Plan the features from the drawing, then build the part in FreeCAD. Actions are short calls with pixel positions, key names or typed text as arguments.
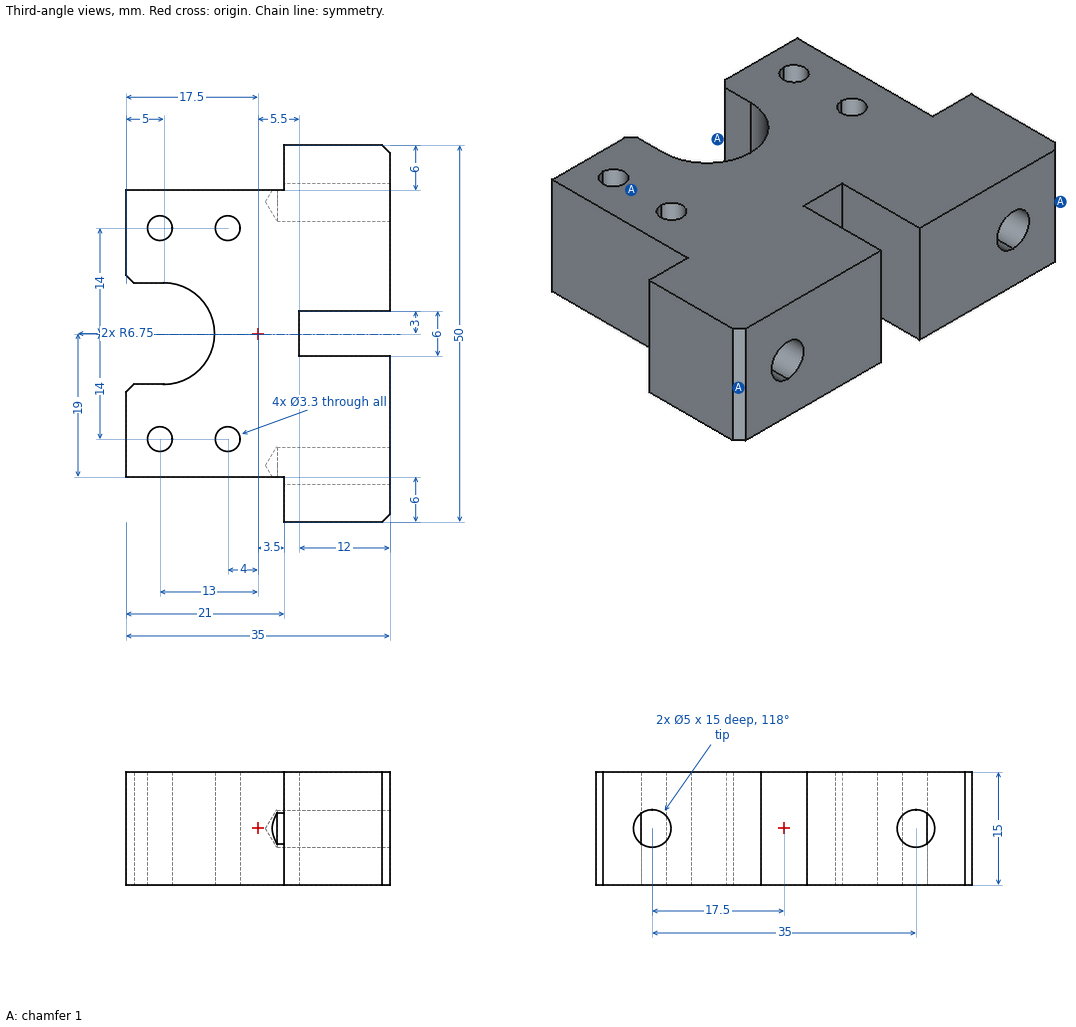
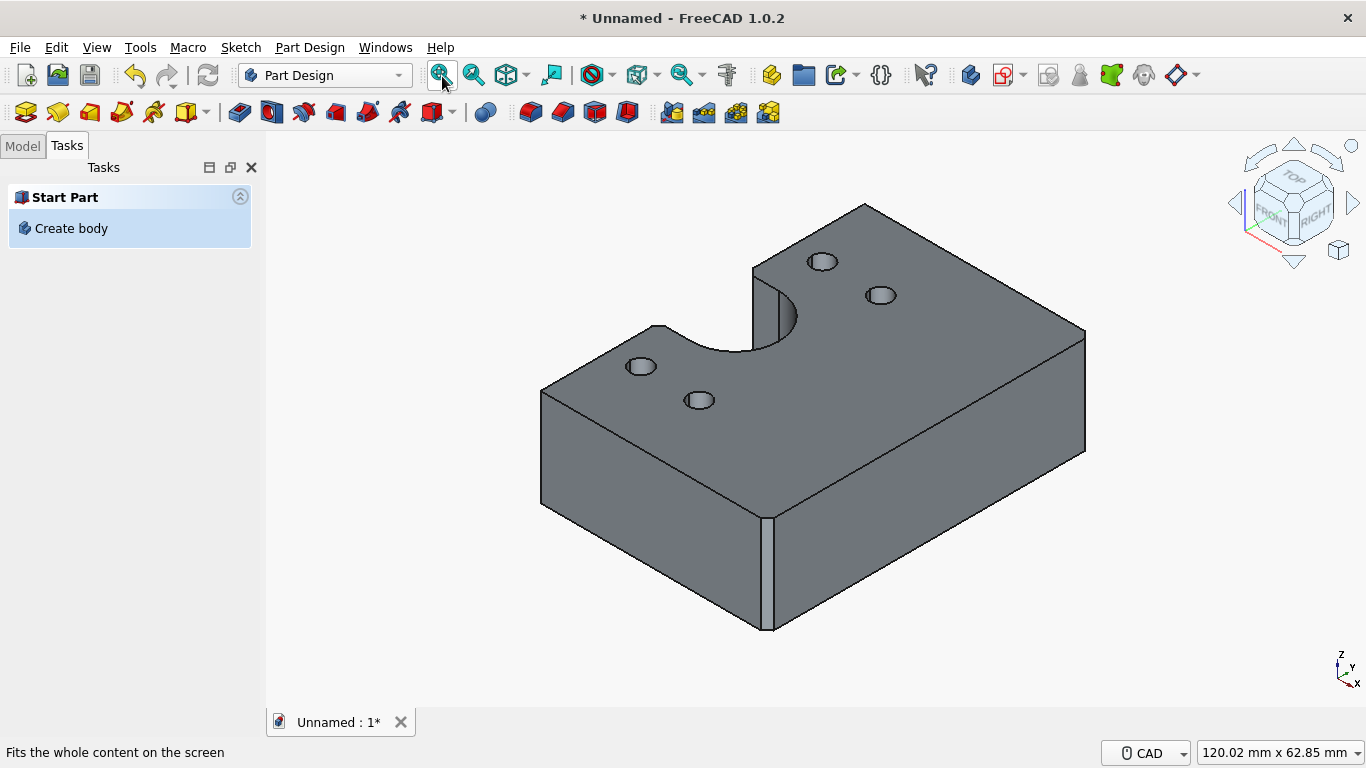
click(1018, 432)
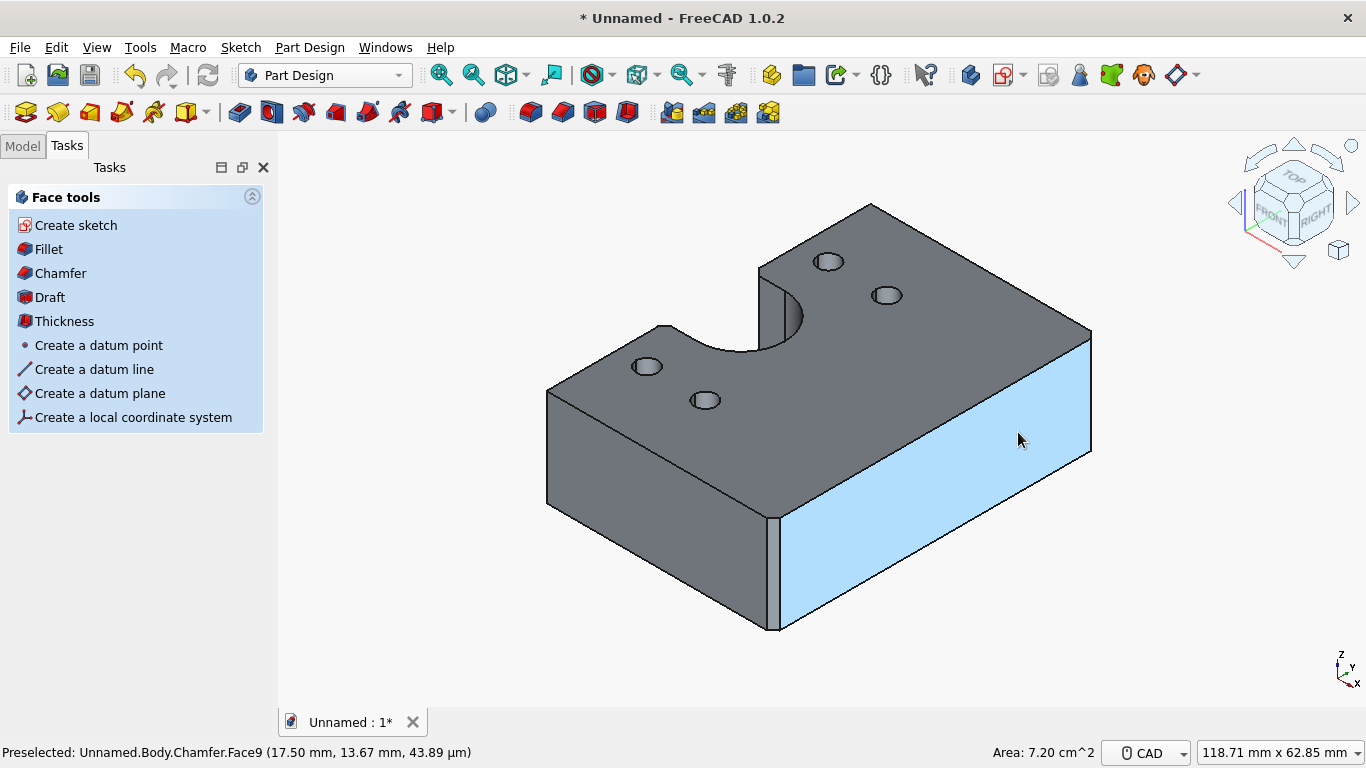
click(1004, 76)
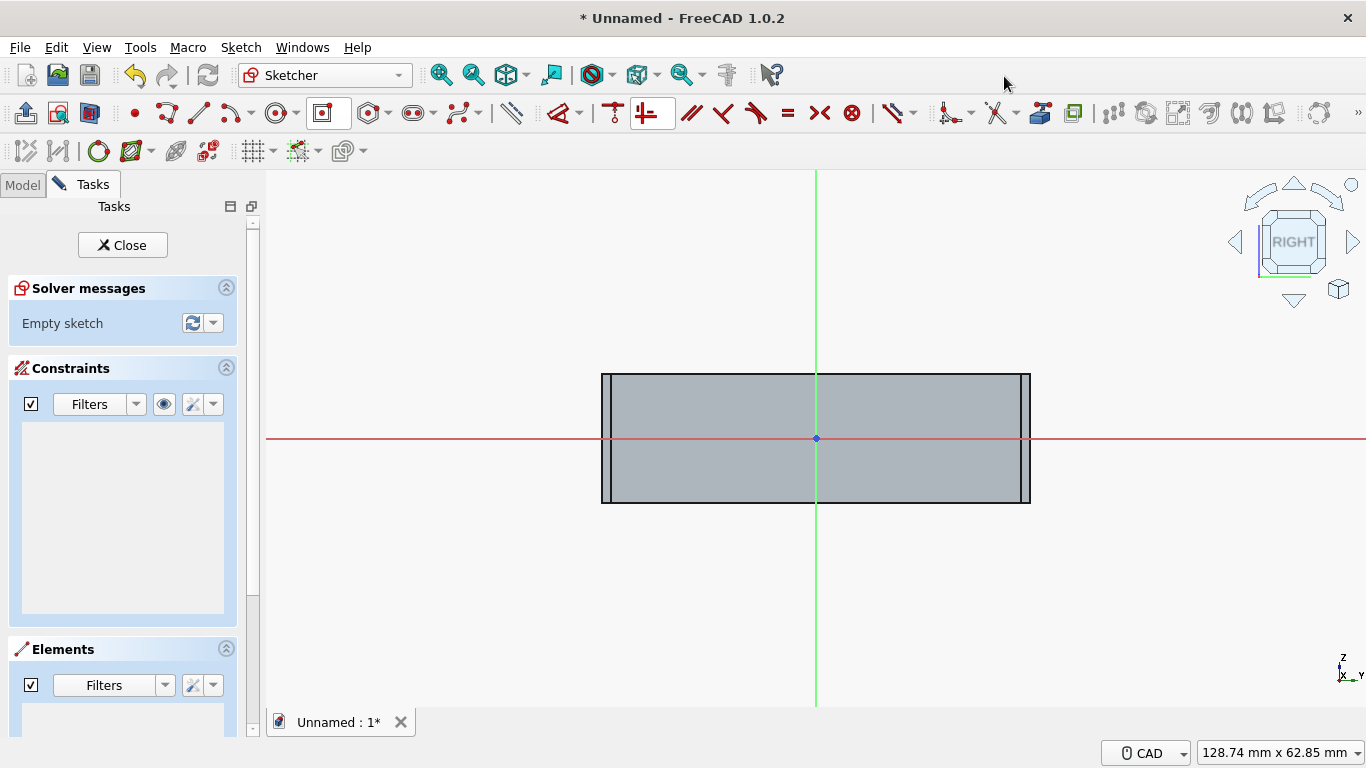
scroll(899, 438, up, 3)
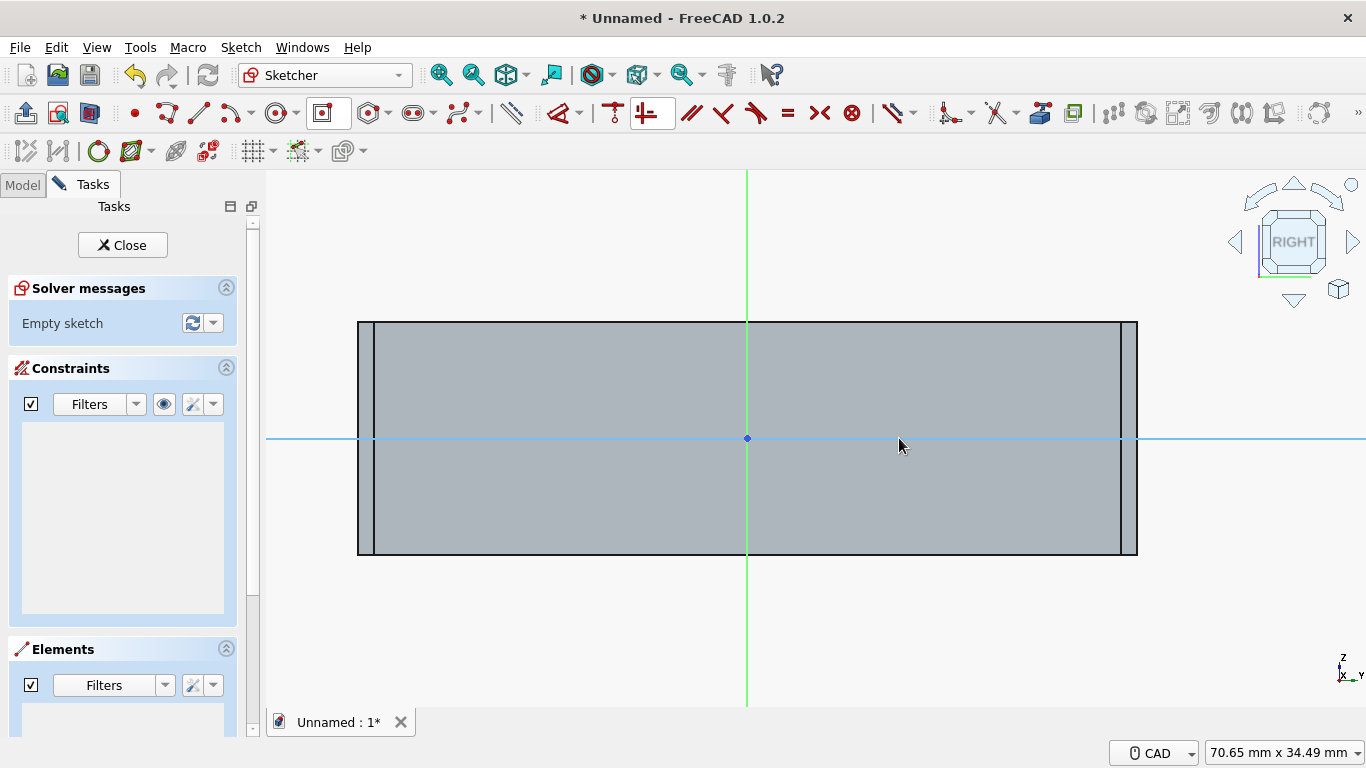
click(276, 114)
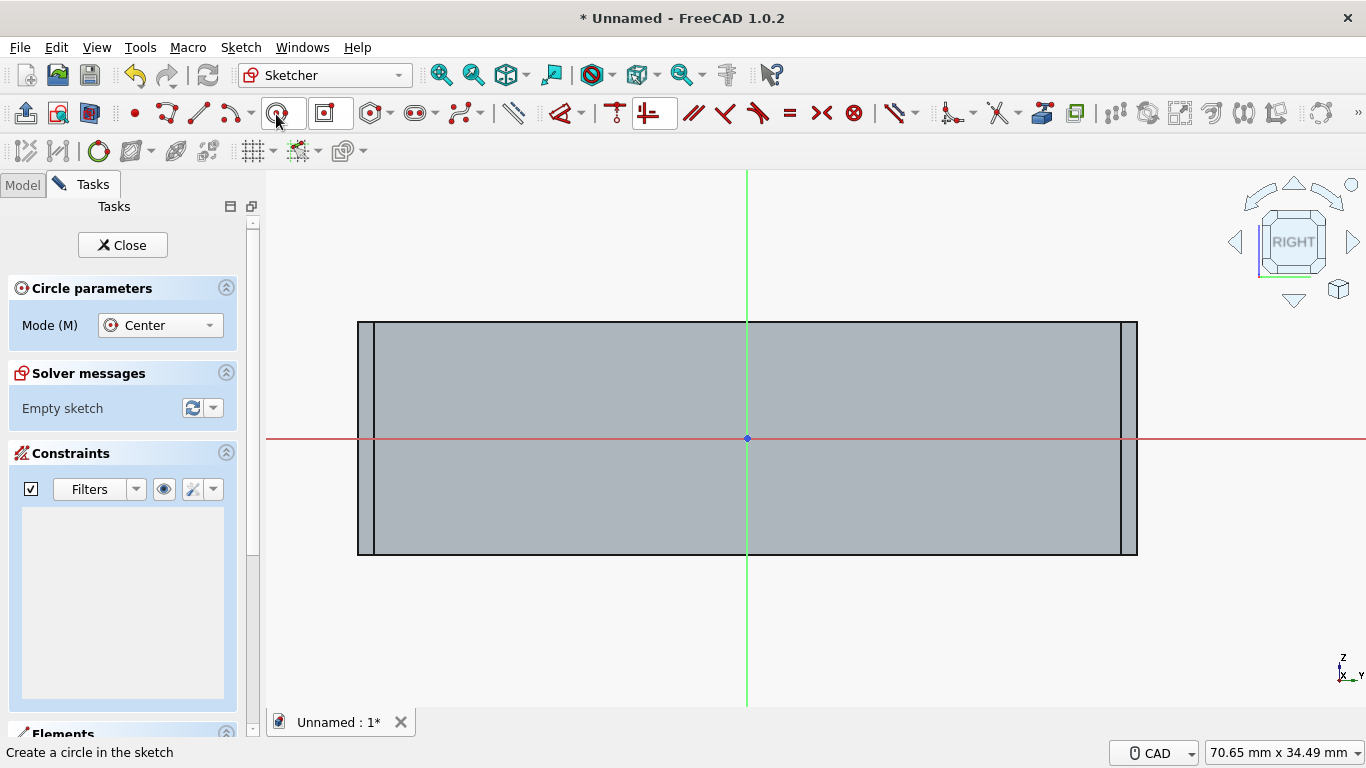
click(475, 438)
move(502, 411)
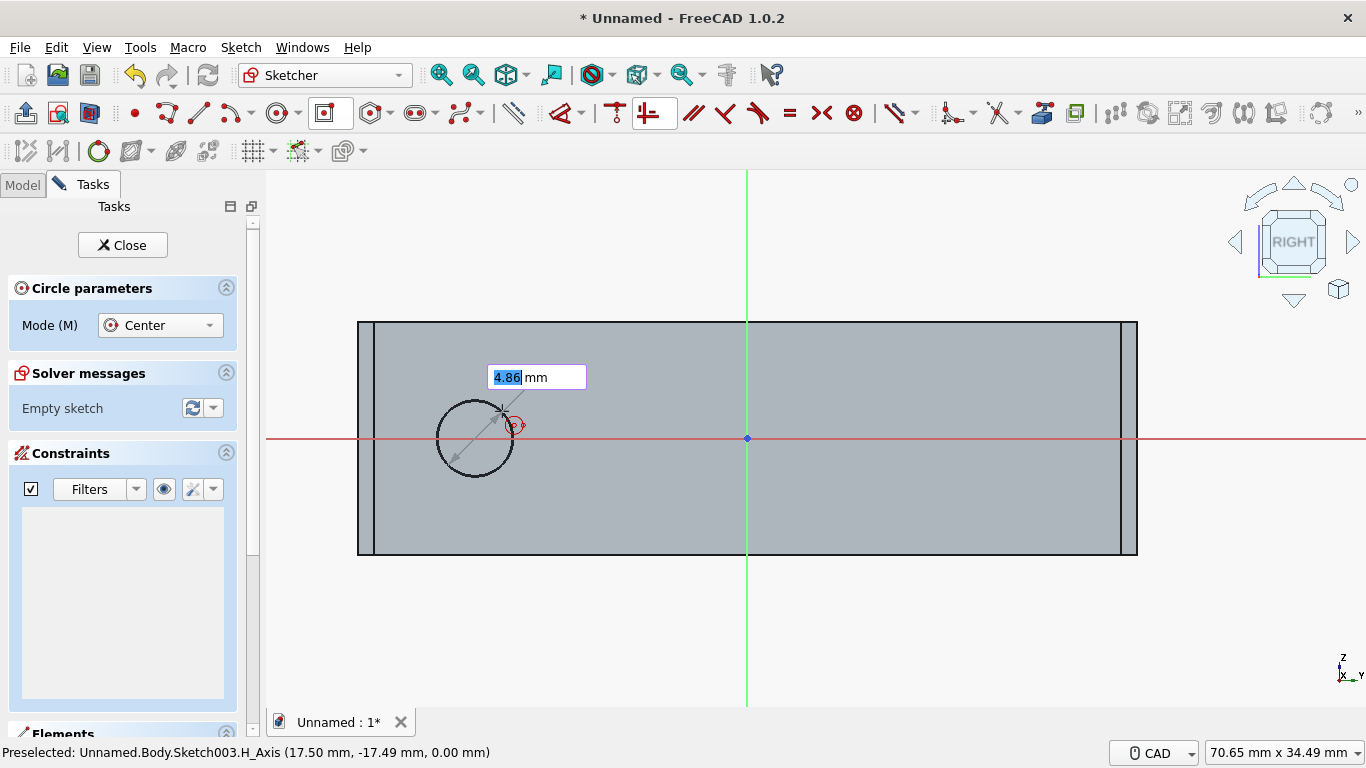
text(5)
key(Return)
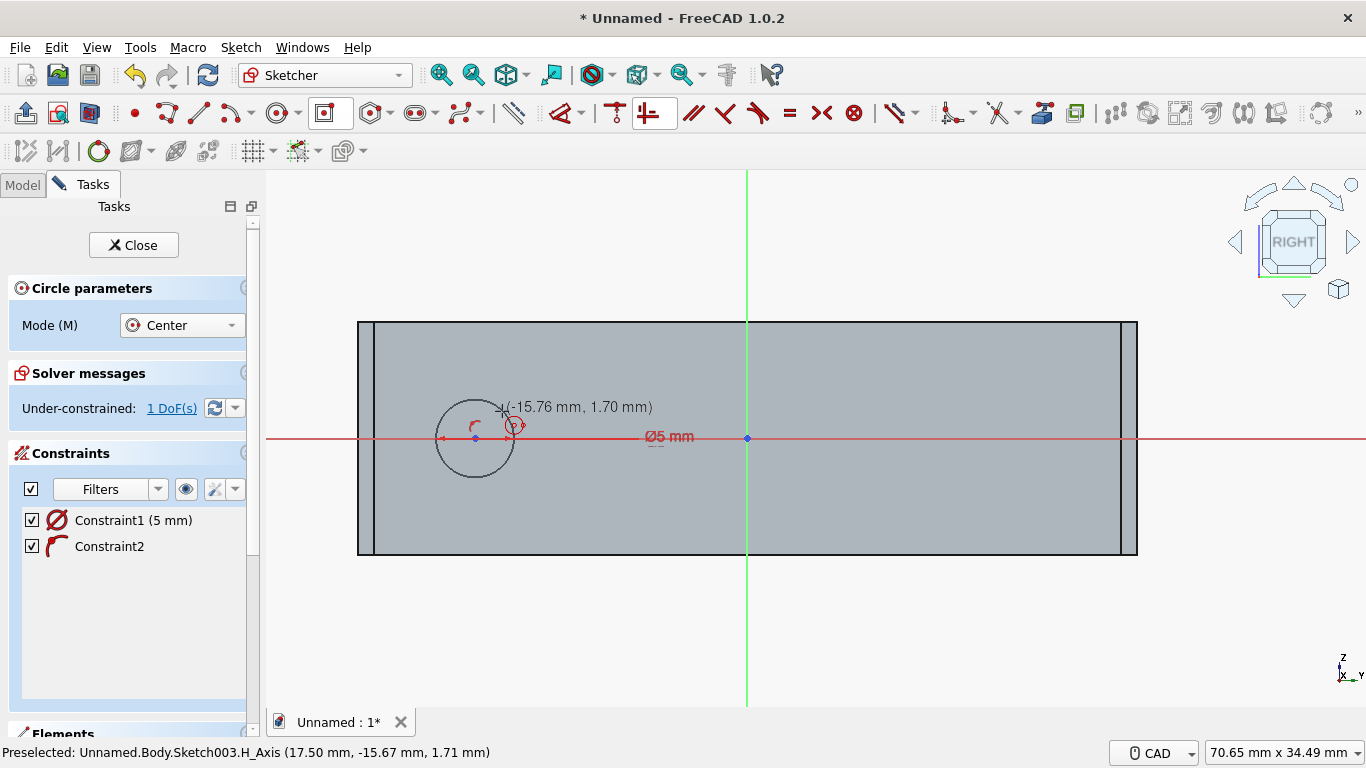
click(1020, 438)
move(1047, 411)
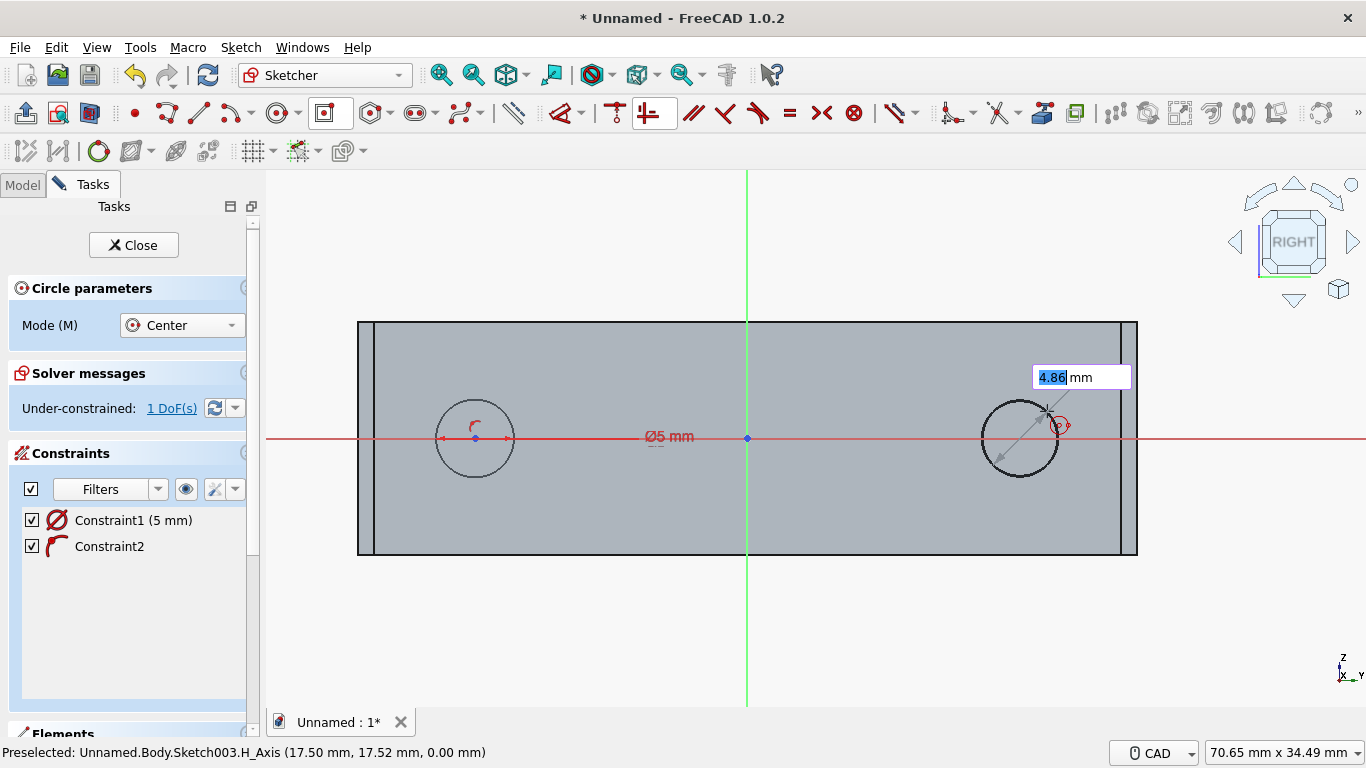
text(5)
key(Return)
key(Escape)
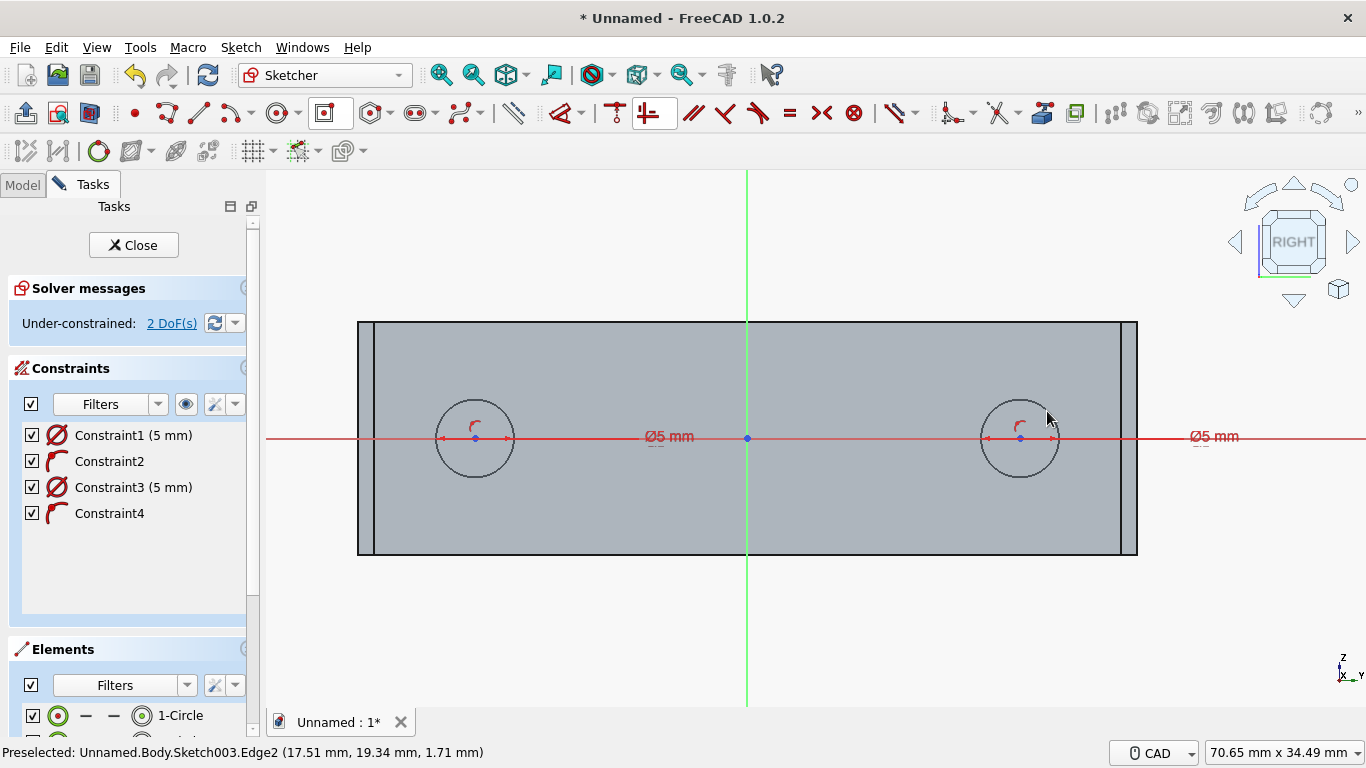
click(560, 114)